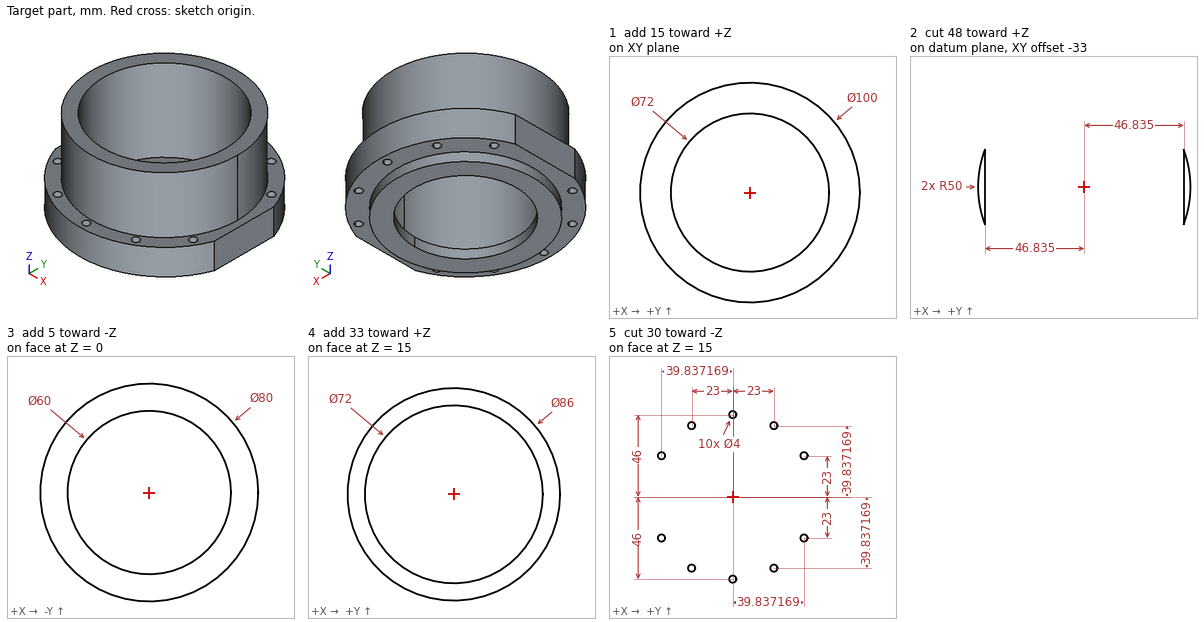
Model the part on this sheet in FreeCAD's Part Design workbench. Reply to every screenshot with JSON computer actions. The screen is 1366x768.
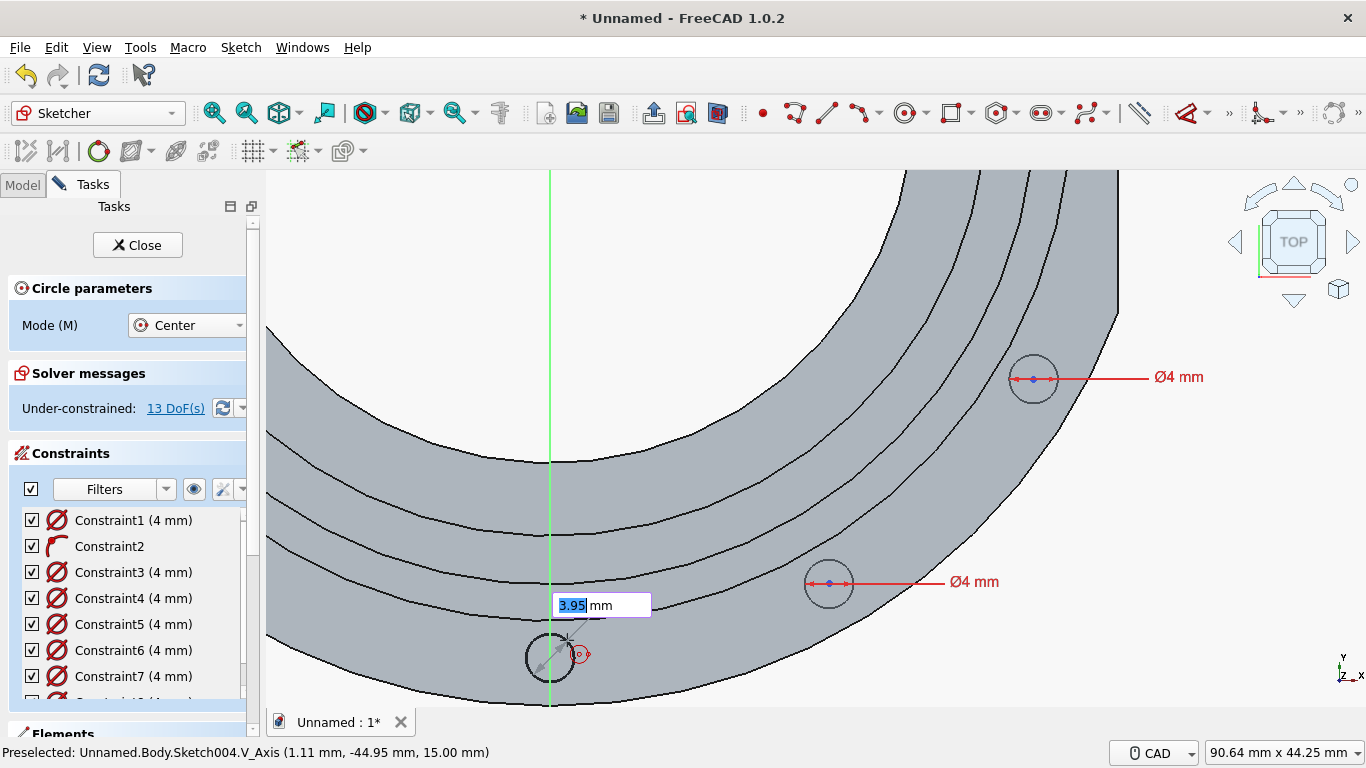
{"action": "type", "text": "4"}
{"action": "key", "text": "Return"}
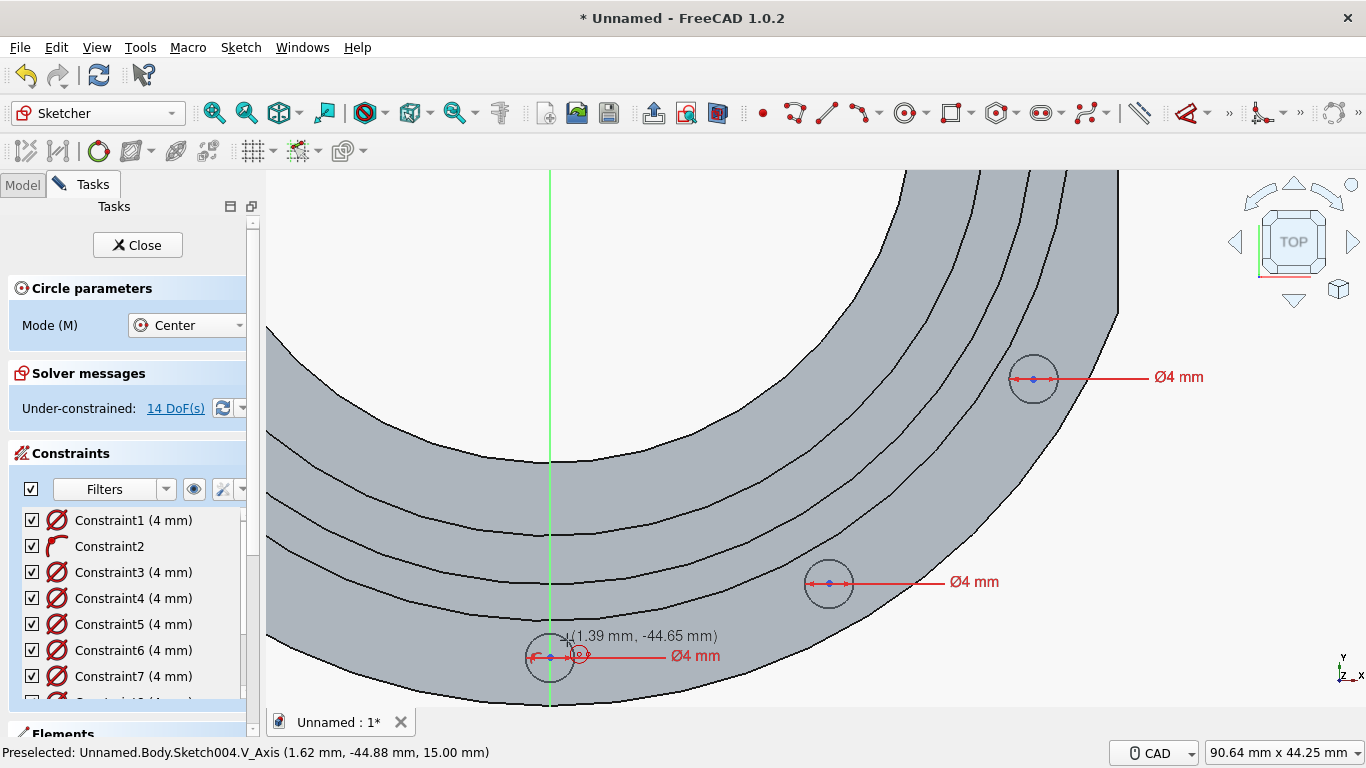
{"action": "scroll", "coordinate": [833, 585], "scroll_direction": "down", "scroll_amount": 6}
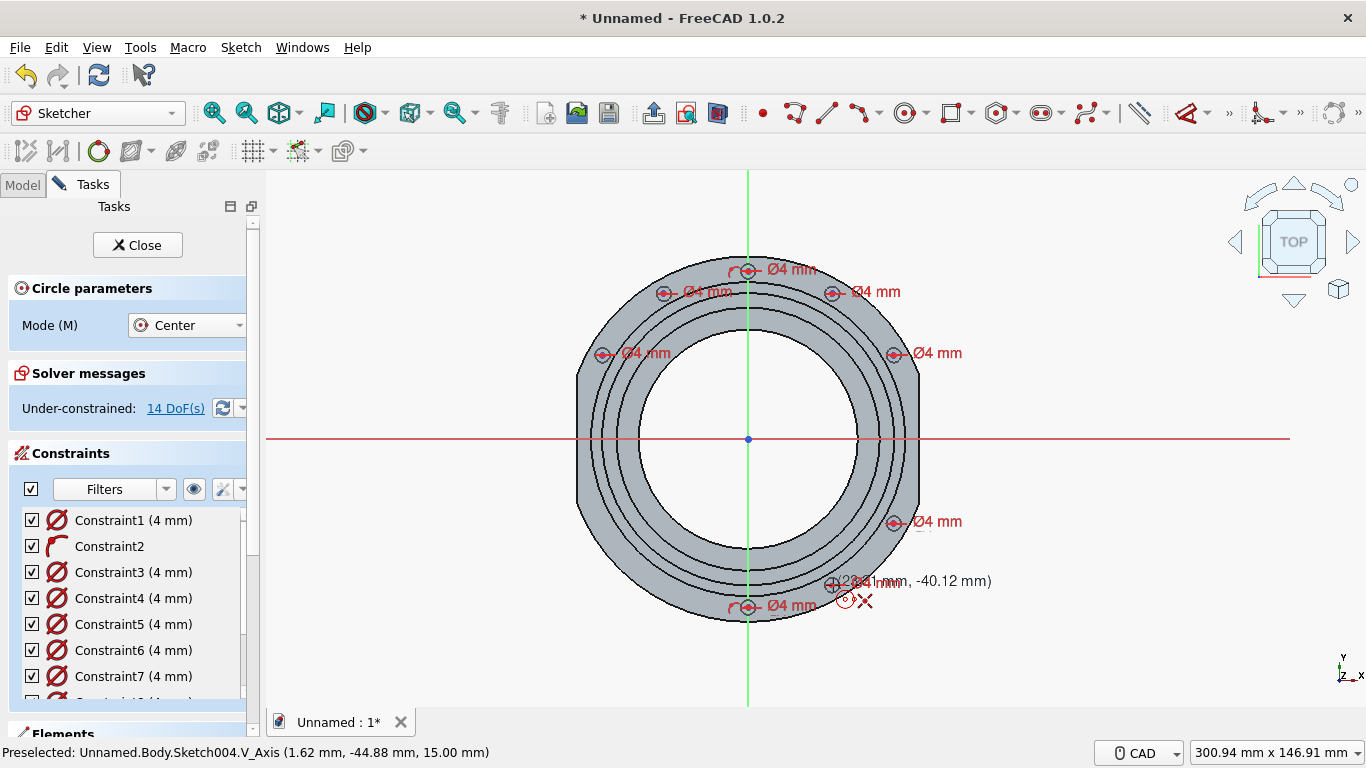
{"action": "scroll", "coordinate": [664, 585], "scroll_direction": "up", "scroll_amount": 6}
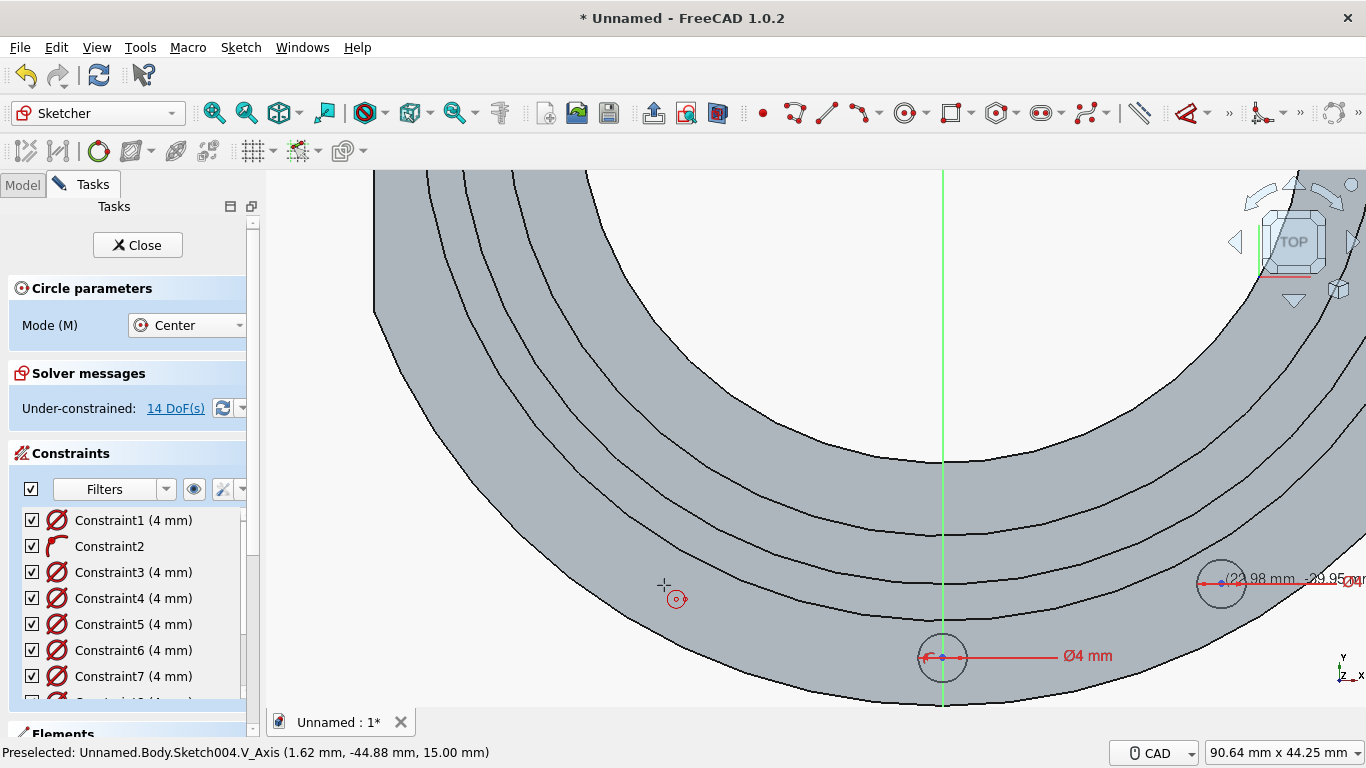
{"action": "left_click", "coordinate": [663, 583]}
{"action": "mouse_move", "coordinate": [681, 565]}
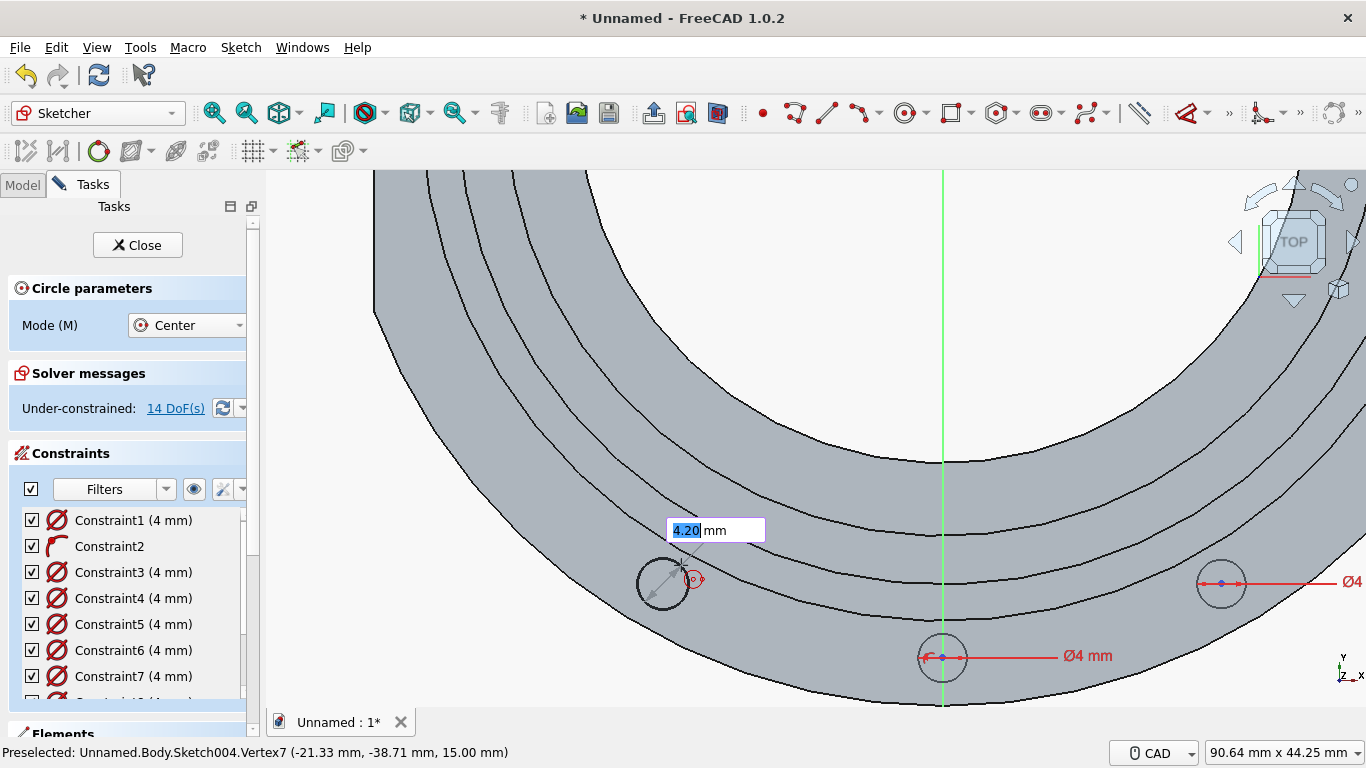
{"action": "type", "text": "4"}
{"action": "key", "text": "Return"}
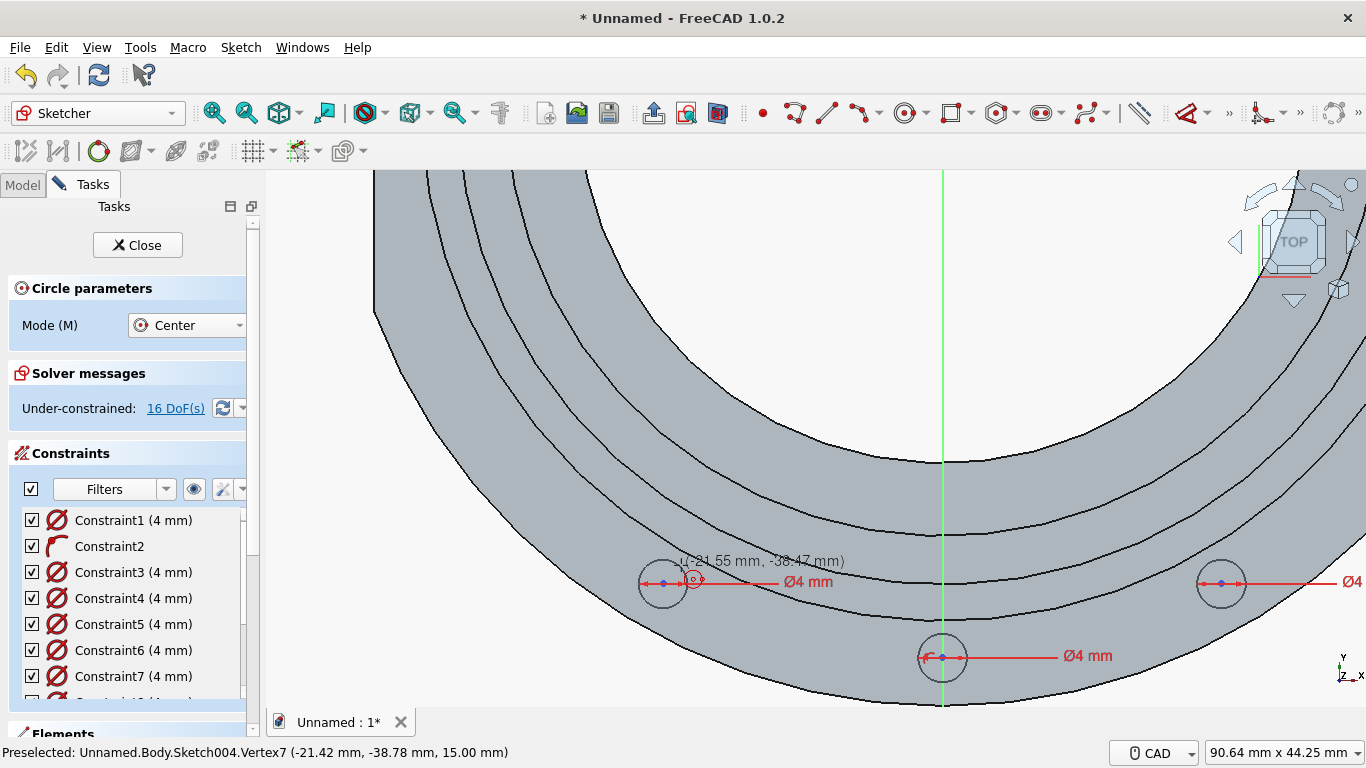
{"action": "left_click", "coordinate": [459, 378]}
{"action": "mouse_move", "coordinate": [476, 361]}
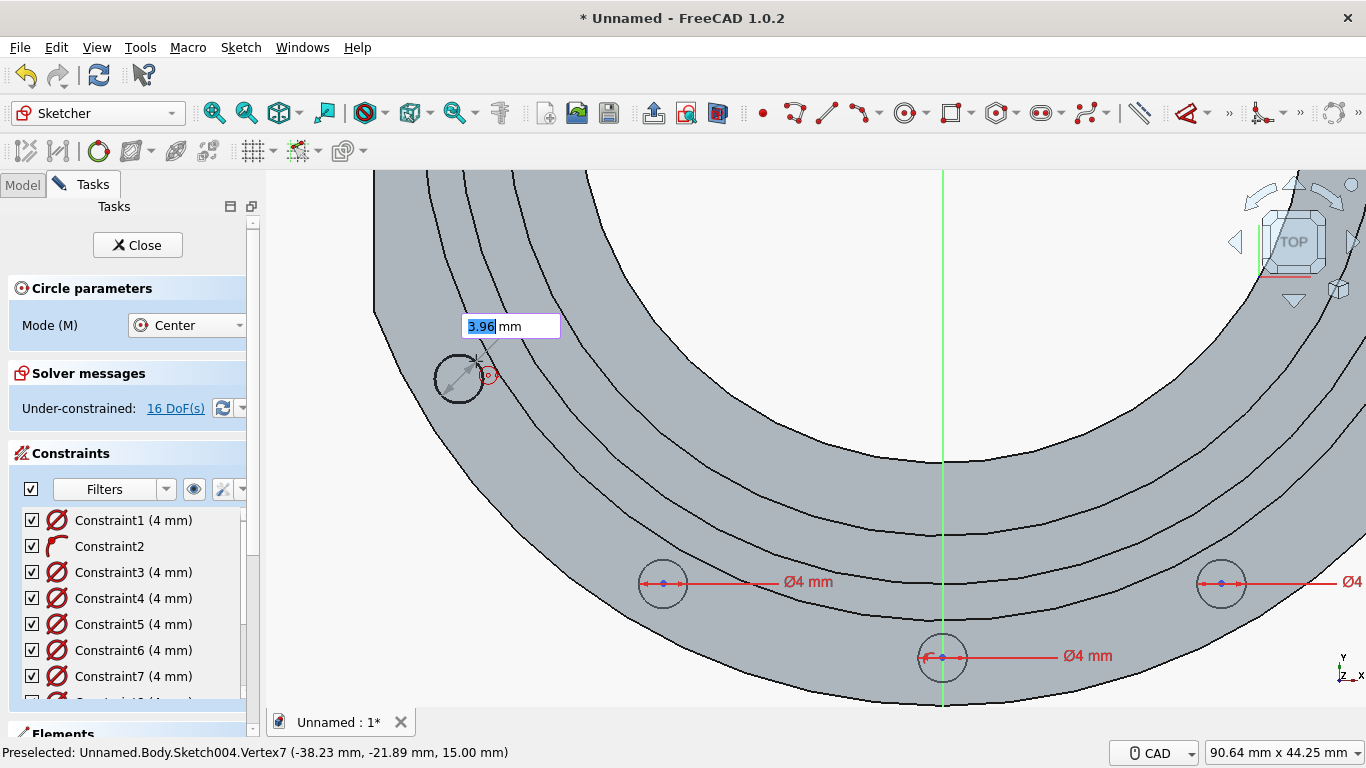
{"action": "type", "text": "4"}
{"action": "key", "text": "Return"}
{"action": "key", "text": "Escape"}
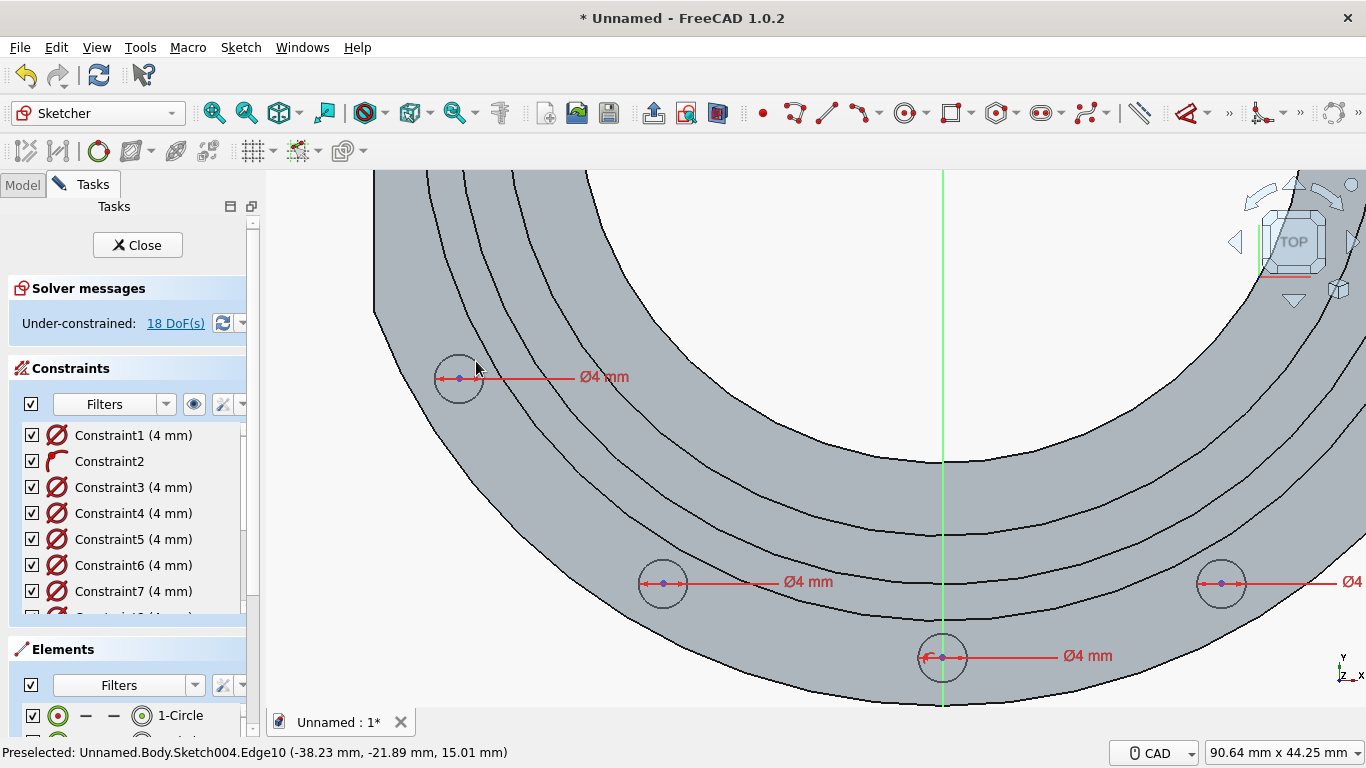
{"action": "scroll", "coordinate": [663, 585], "scroll_direction": "down", "scroll_amount": 6}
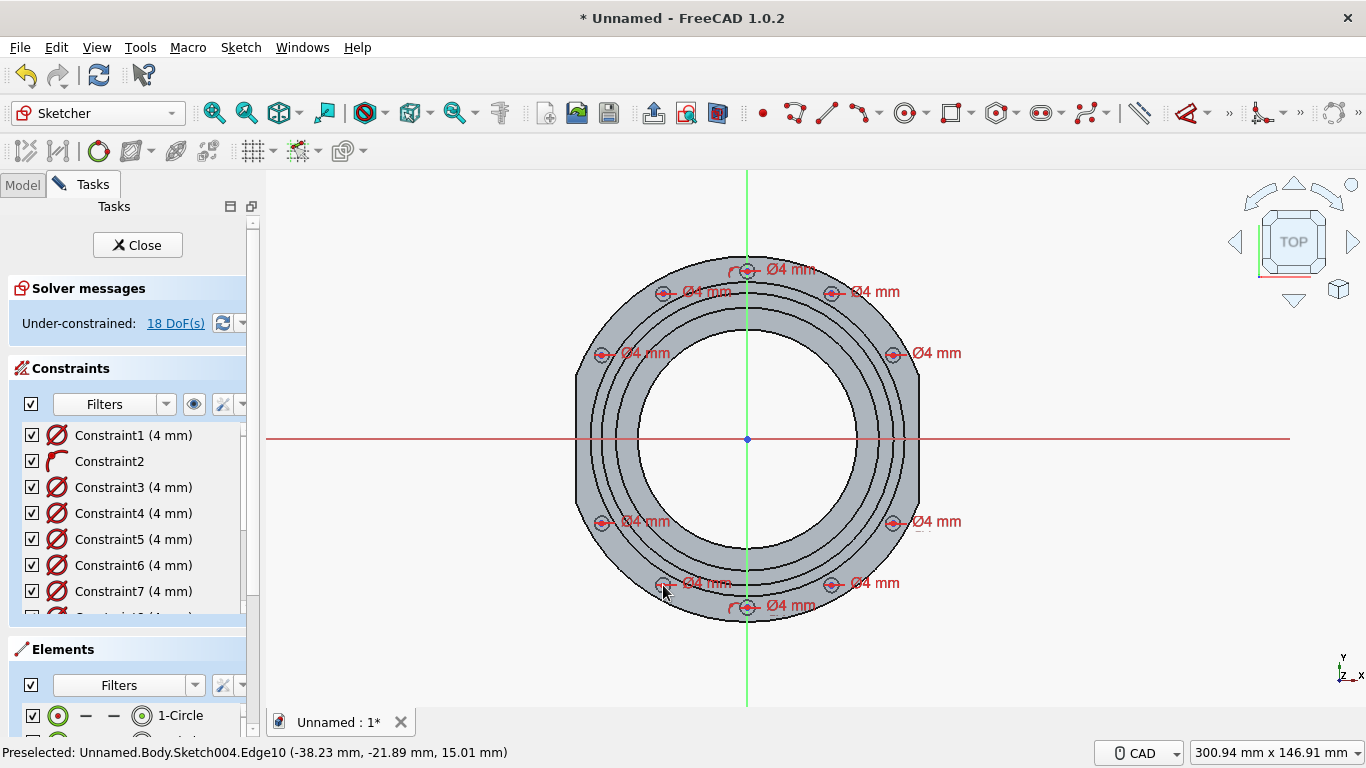
{"action": "left_click", "coordinate": [893, 524]}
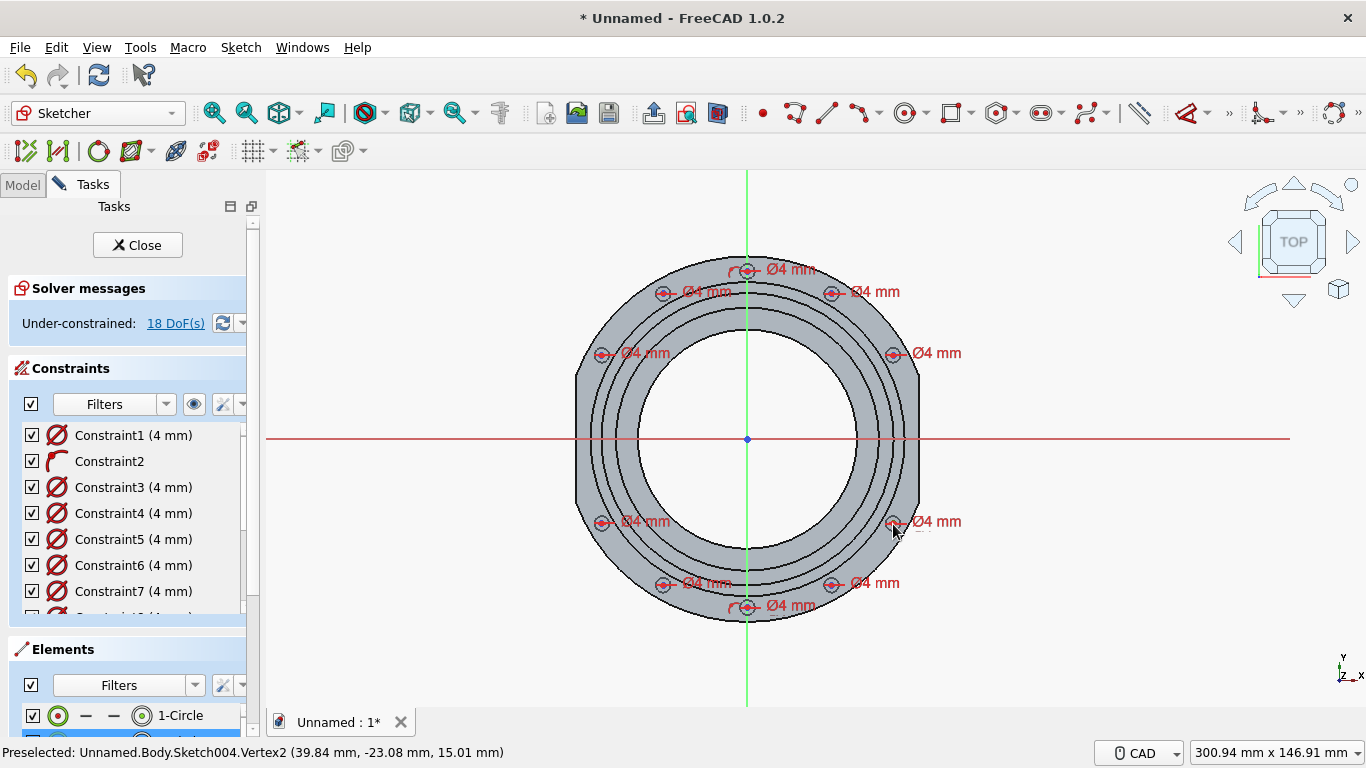
{"action": "left_click", "coordinate": [893, 355]}